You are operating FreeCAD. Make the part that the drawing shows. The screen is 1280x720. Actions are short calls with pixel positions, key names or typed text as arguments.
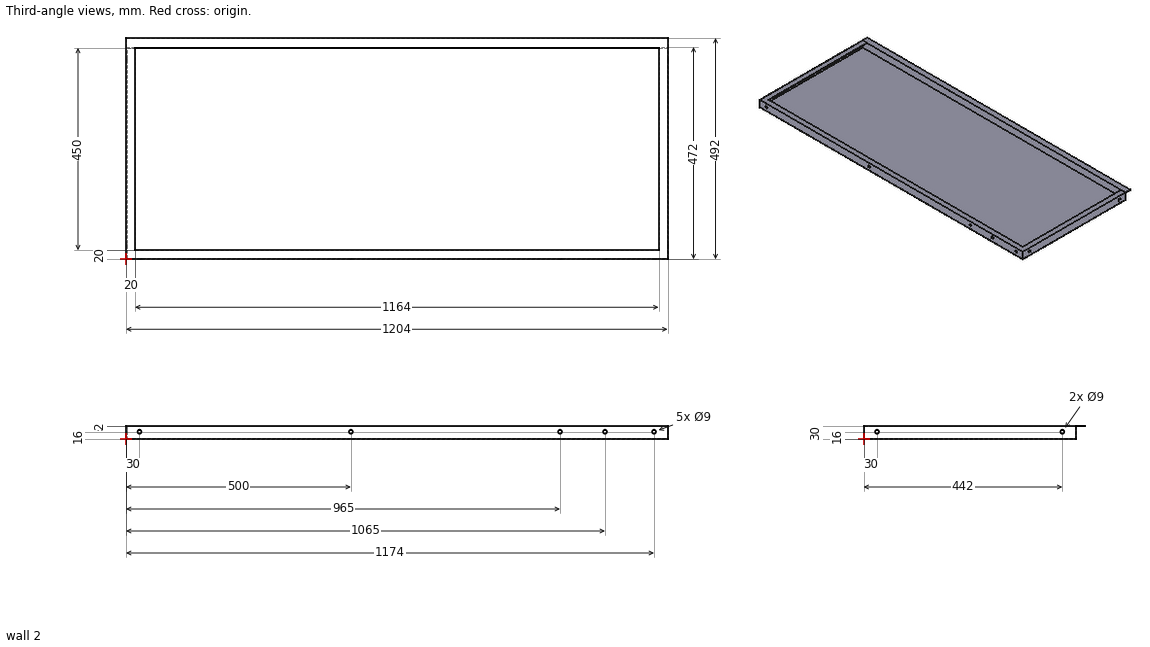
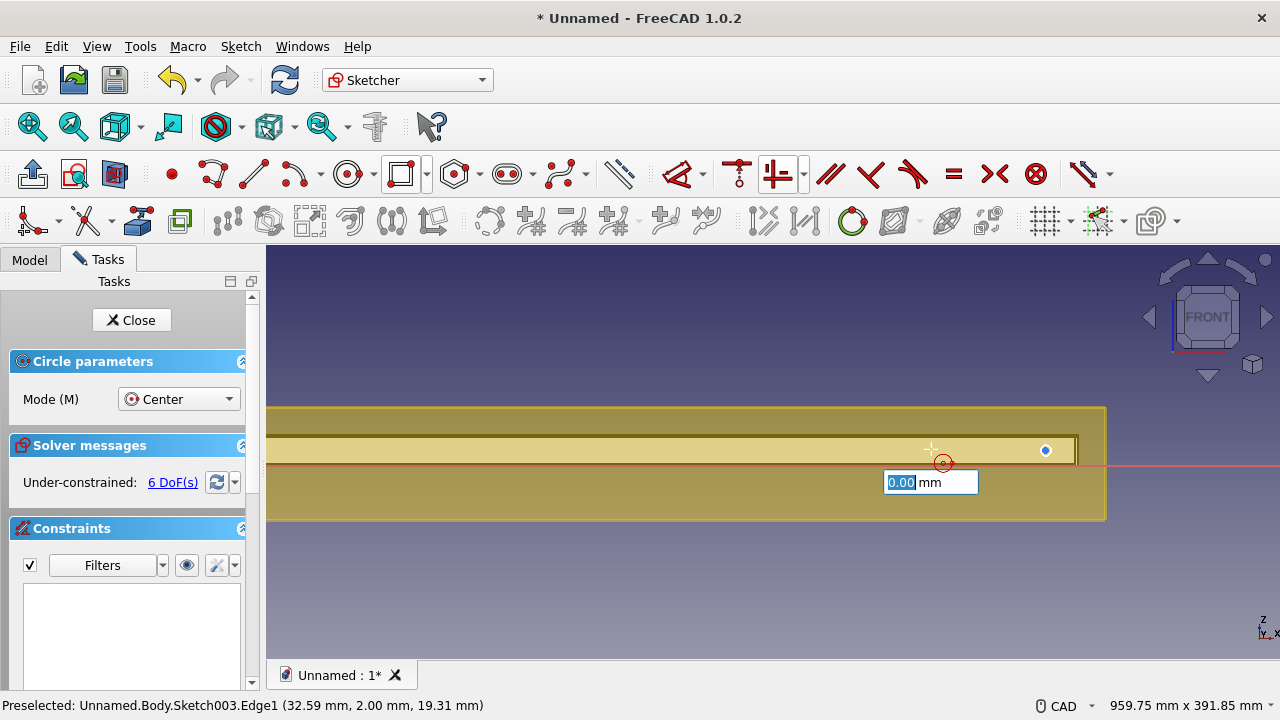
scroll(934, 446, up, 7)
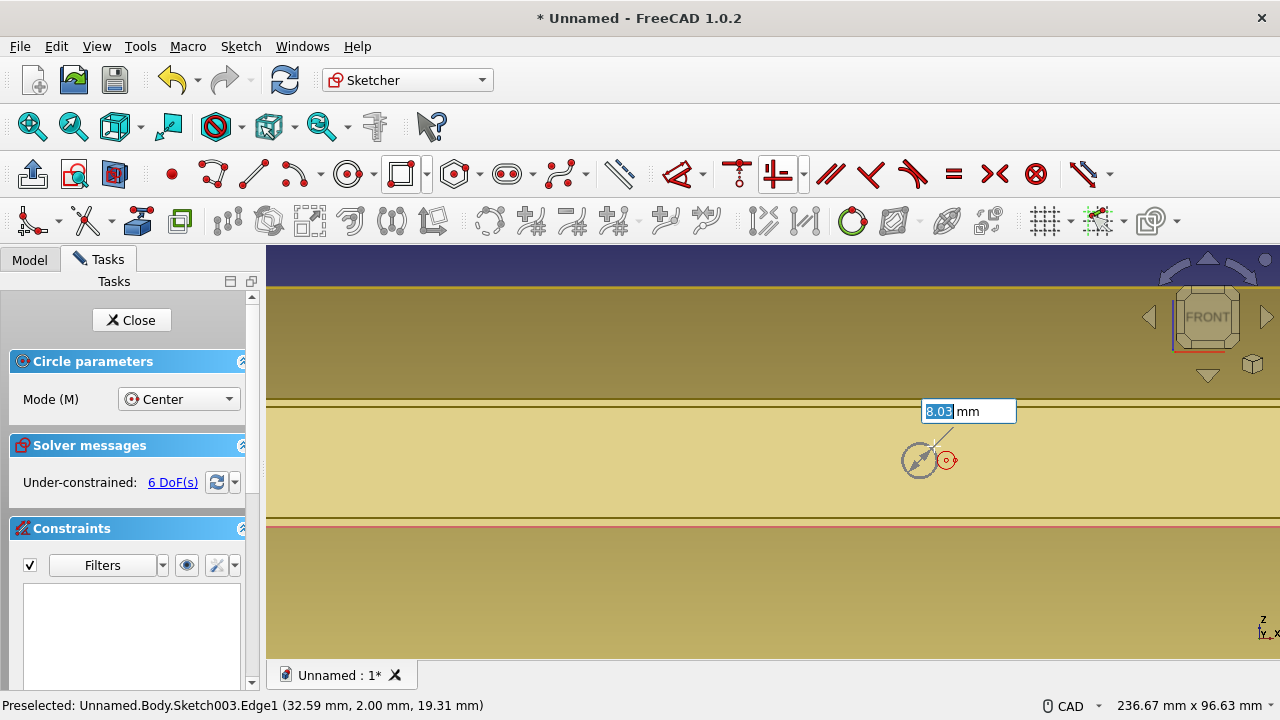
click(932, 445)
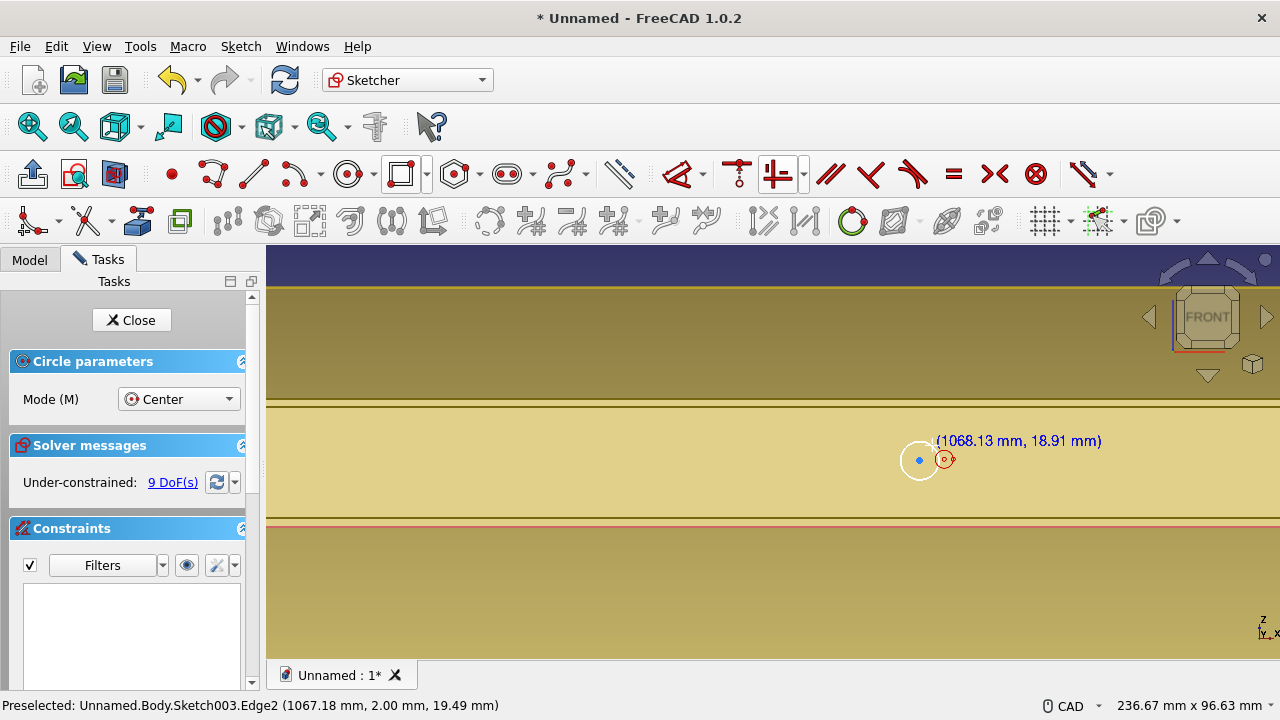
scroll(932, 448, down, 11)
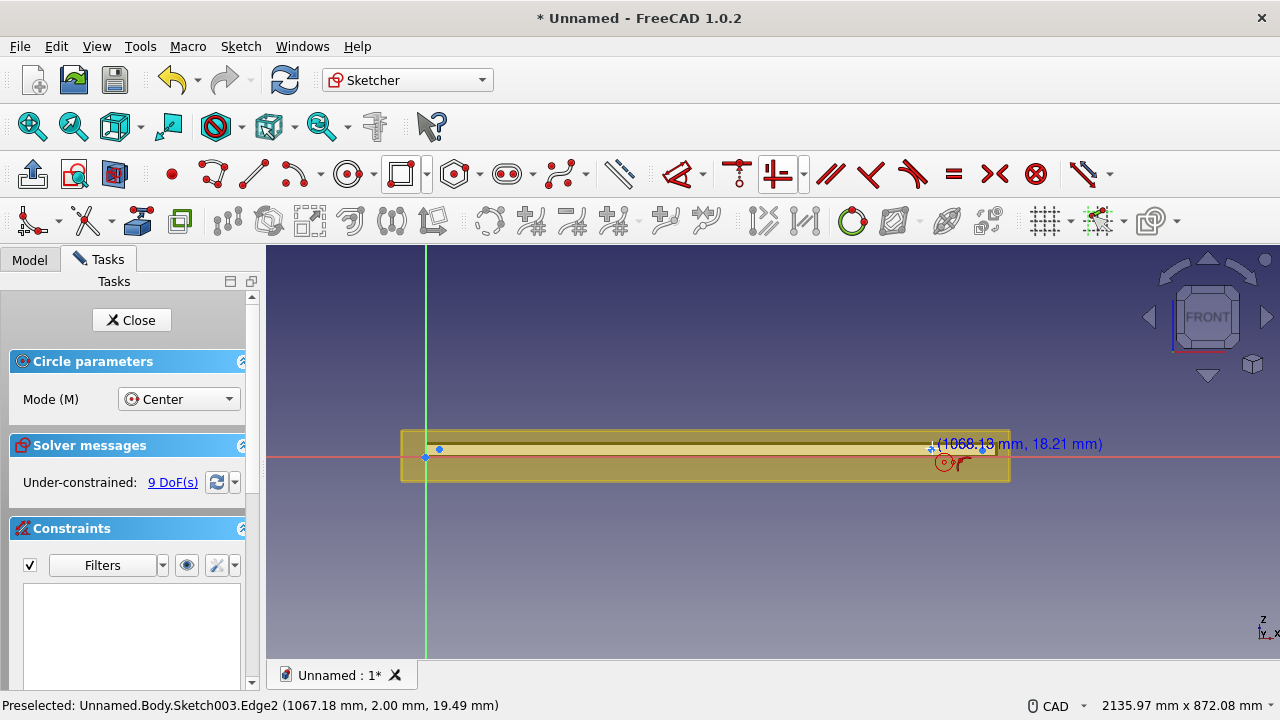
scroll(884, 450, up, 4)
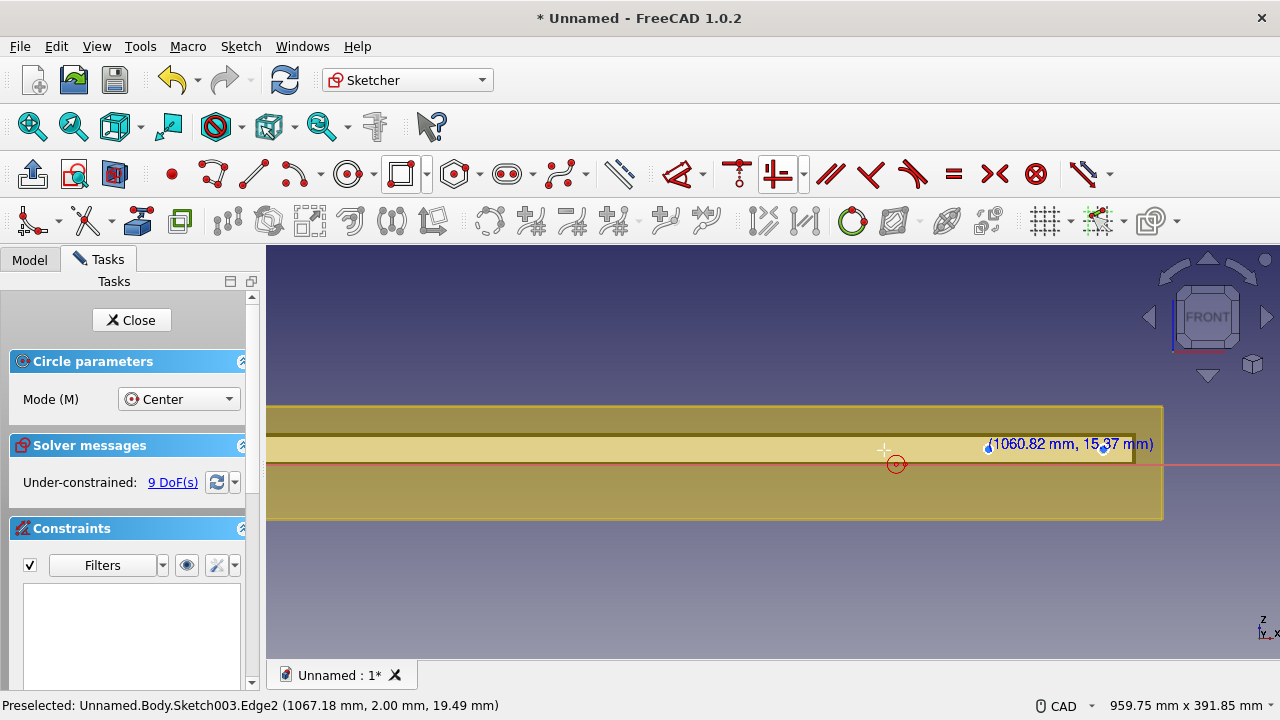
click(882, 448)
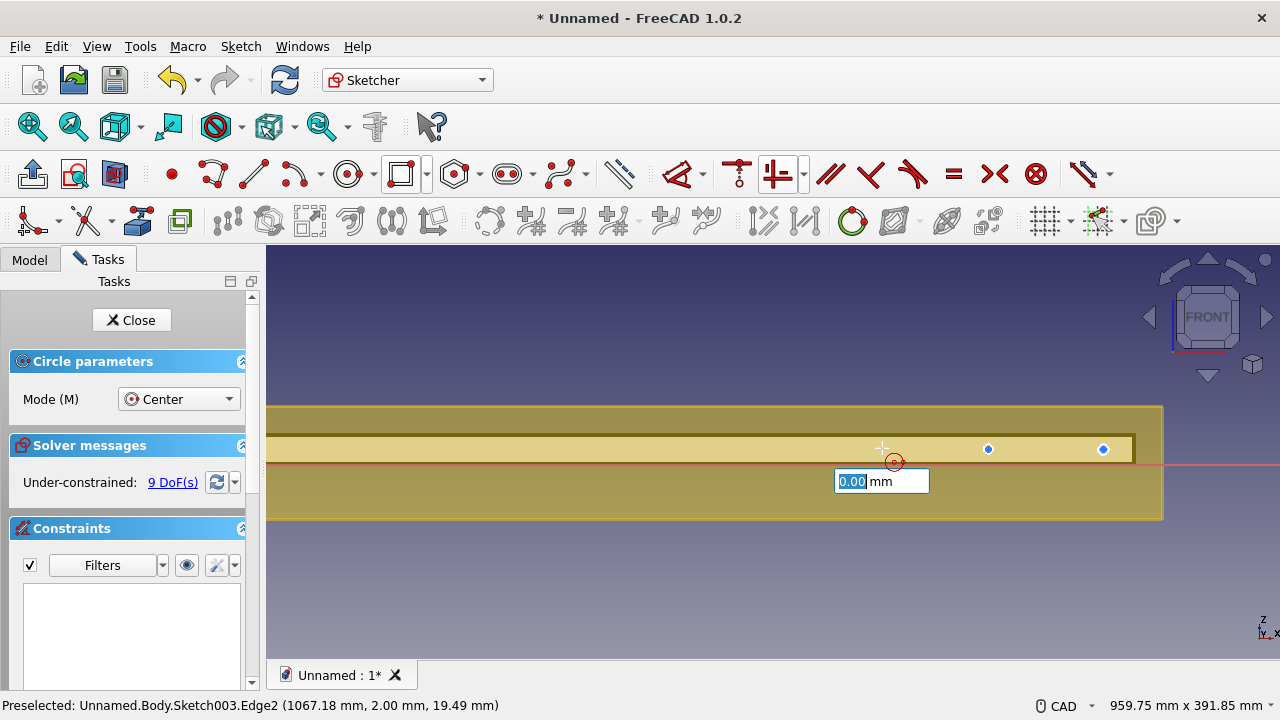
scroll(886, 445, up, 7)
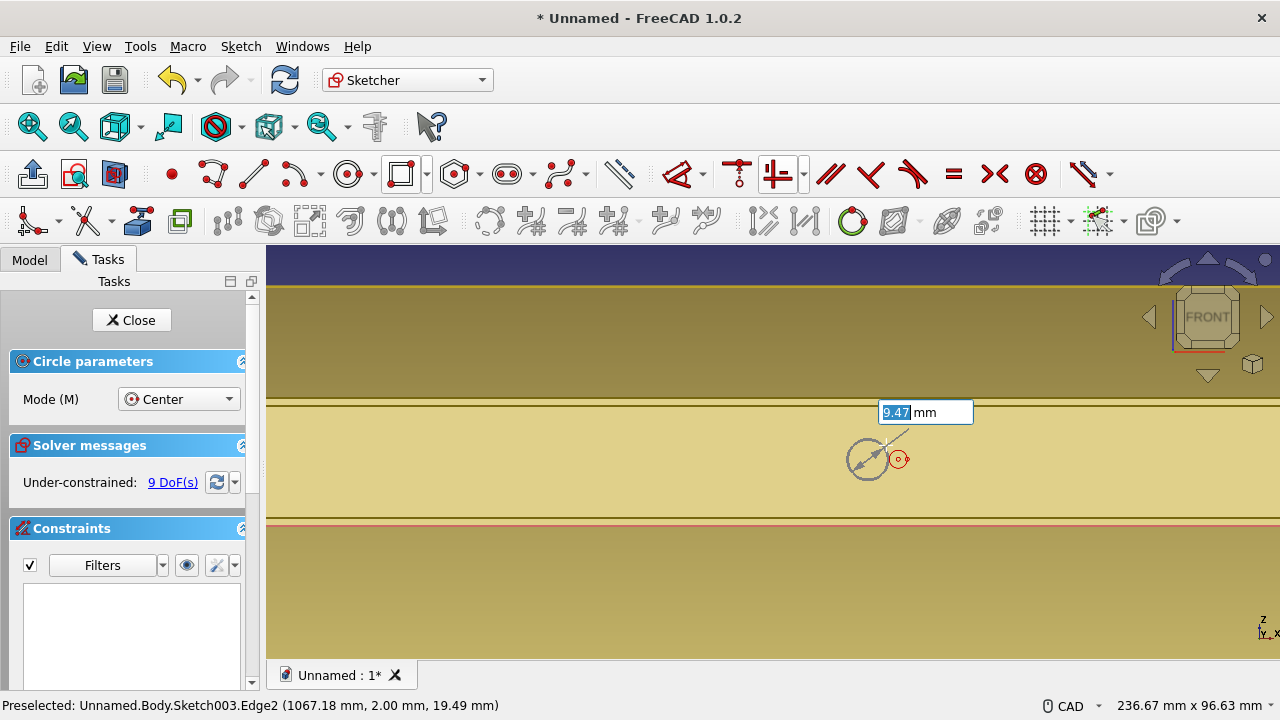
click(883, 444)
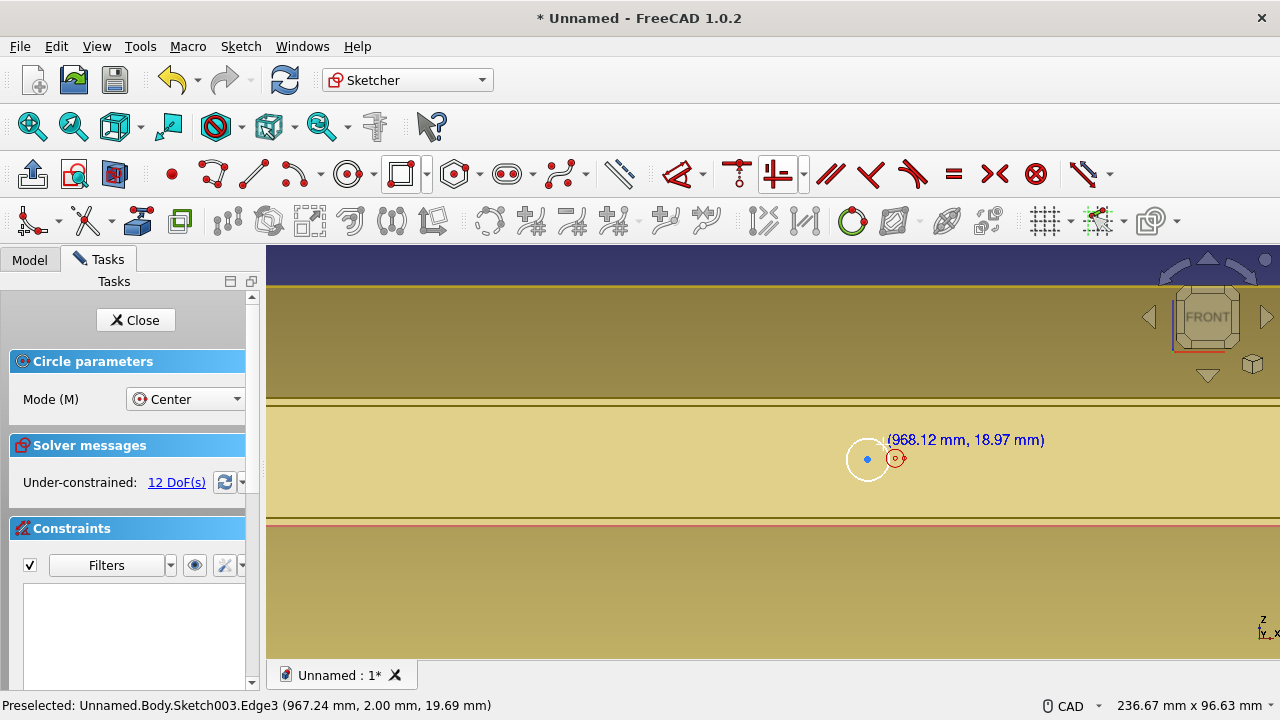
scroll(885, 448, down, 11)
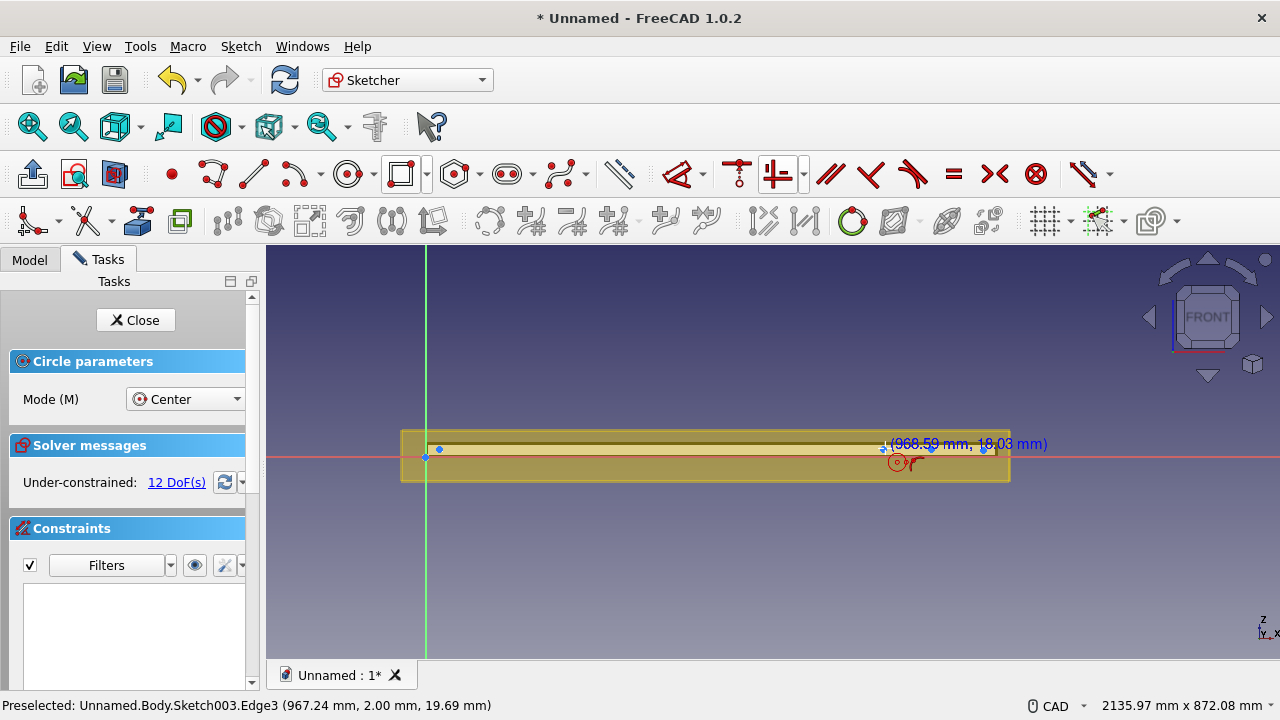
scroll(663, 450, up, 12)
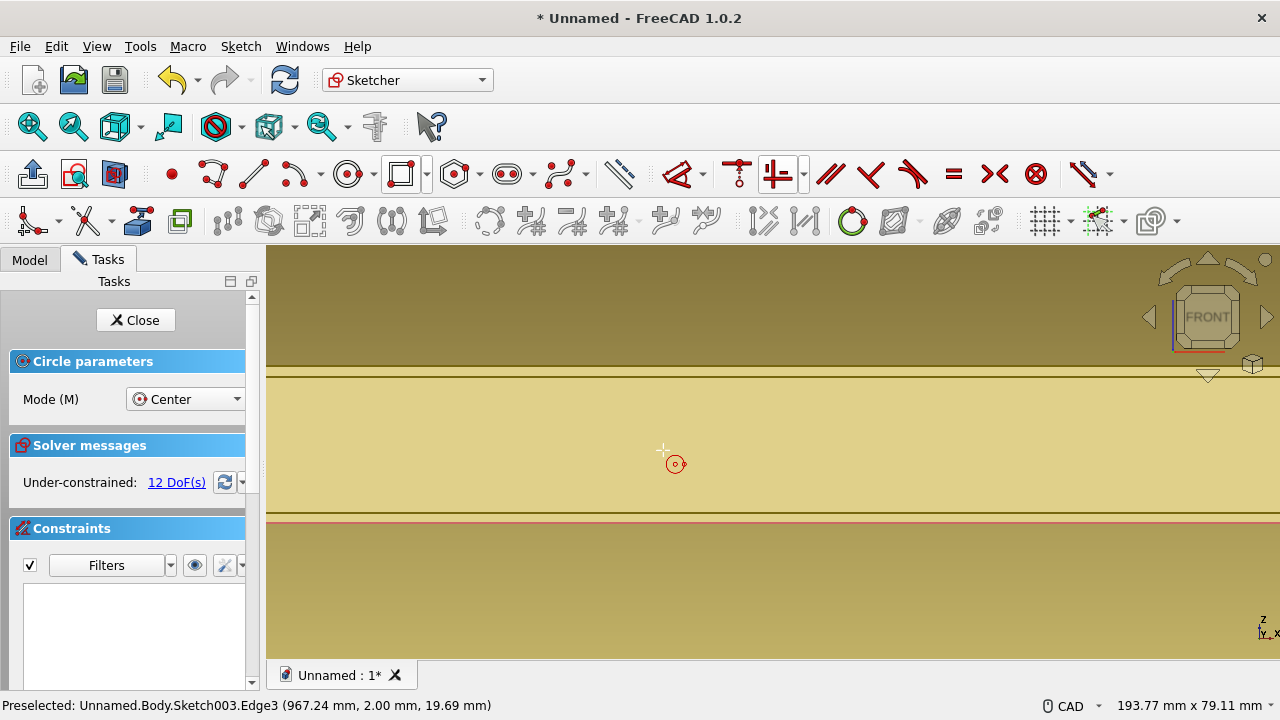
scroll(662, 450, down, 12)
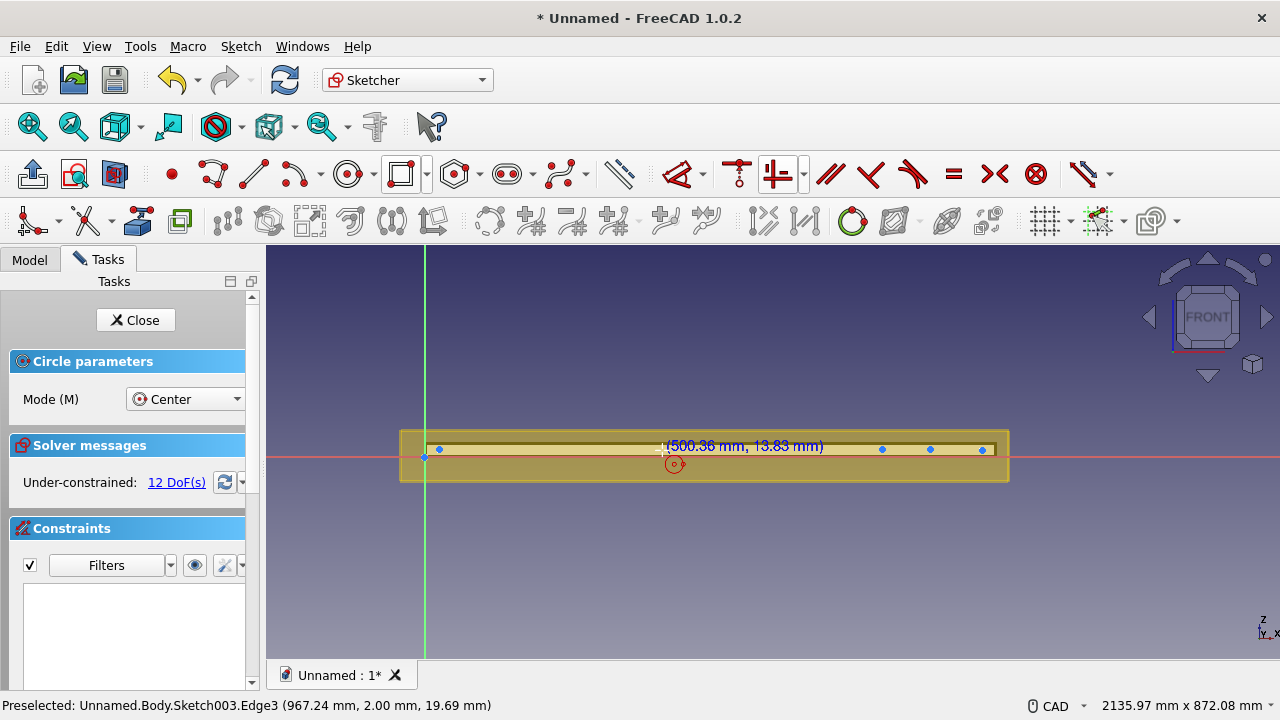
scroll(662, 450, up, 4)